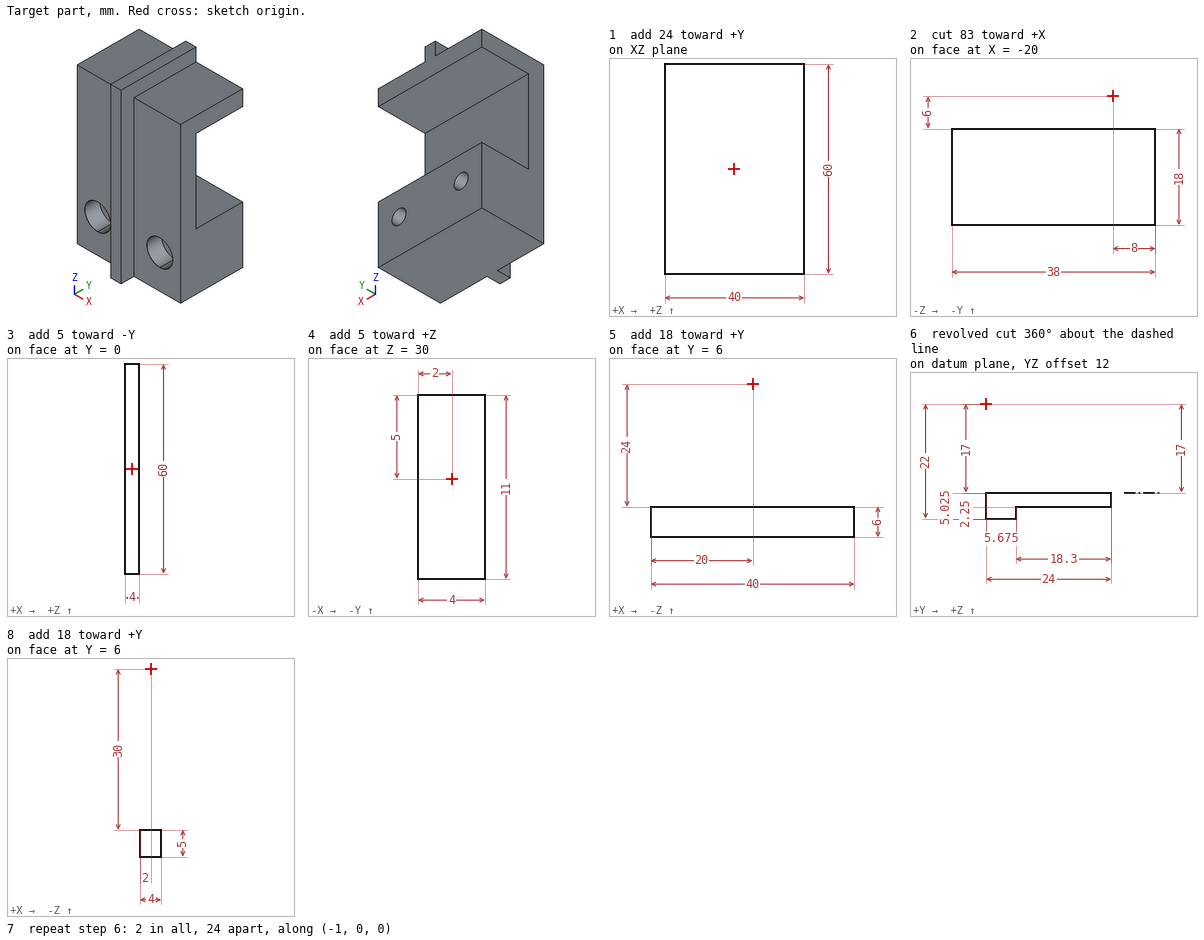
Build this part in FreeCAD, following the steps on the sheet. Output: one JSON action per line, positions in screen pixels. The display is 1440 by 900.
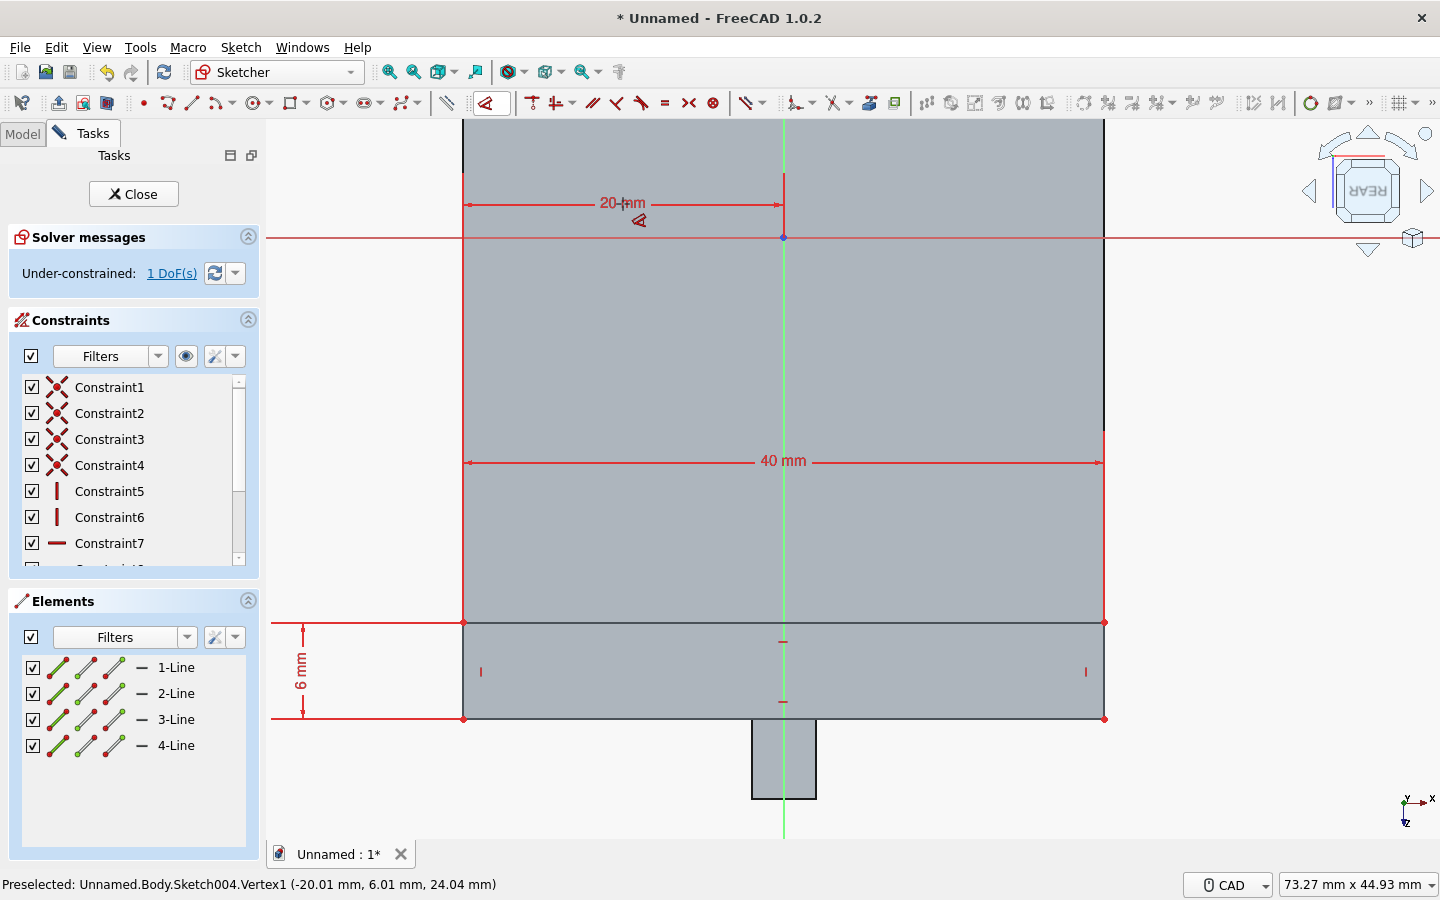
{"action": "left_click", "coordinate": [463, 623]}
{"action": "left_click", "coordinate": [429, 430]}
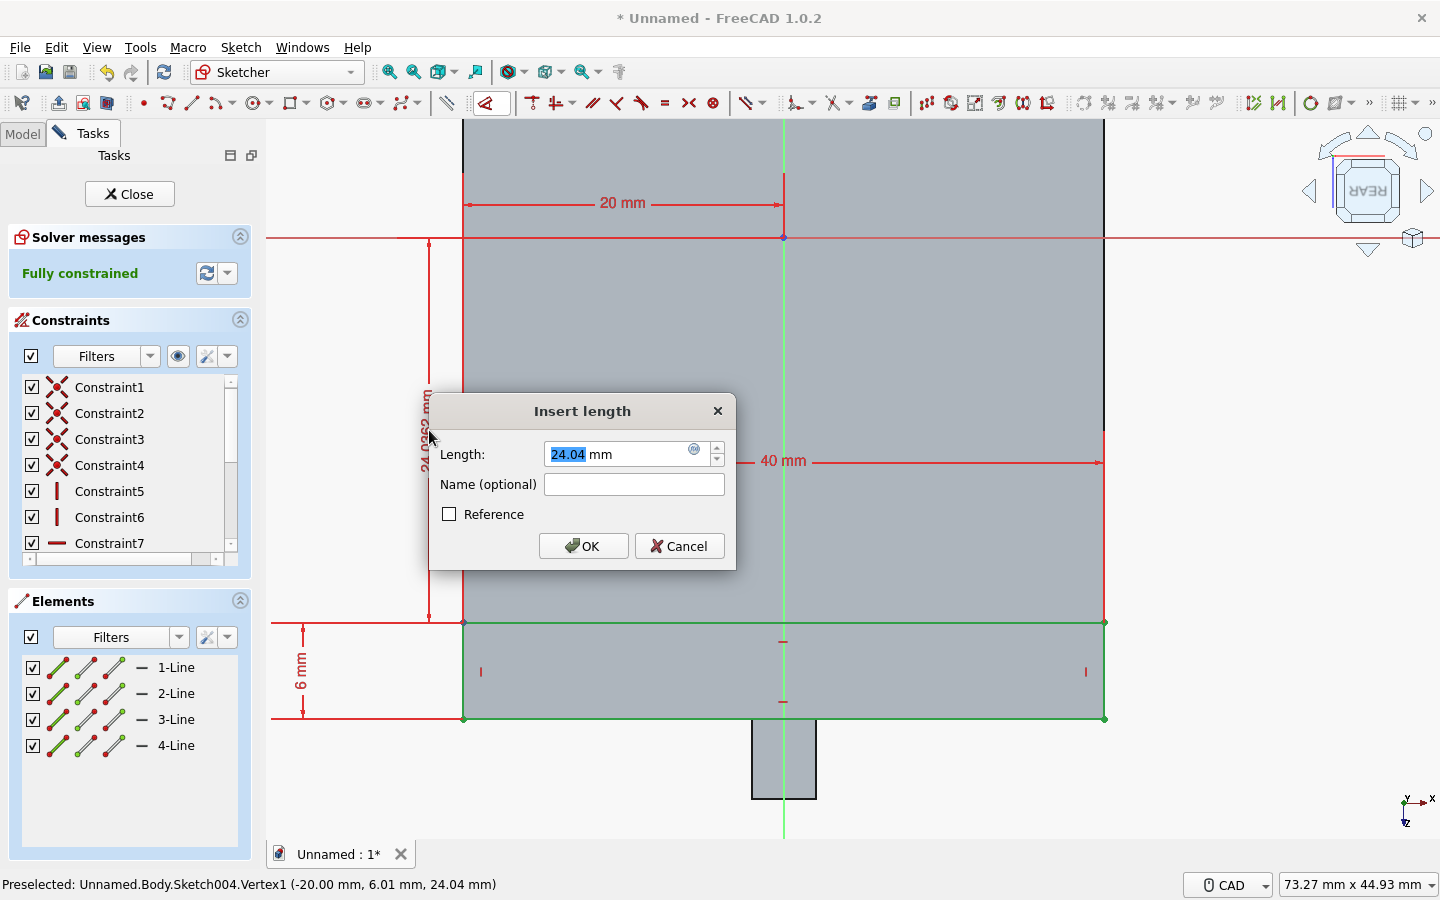
{"action": "type", "text": "24"}
{"action": "key", "text": "Return"}
{"action": "key", "text": "Escape"}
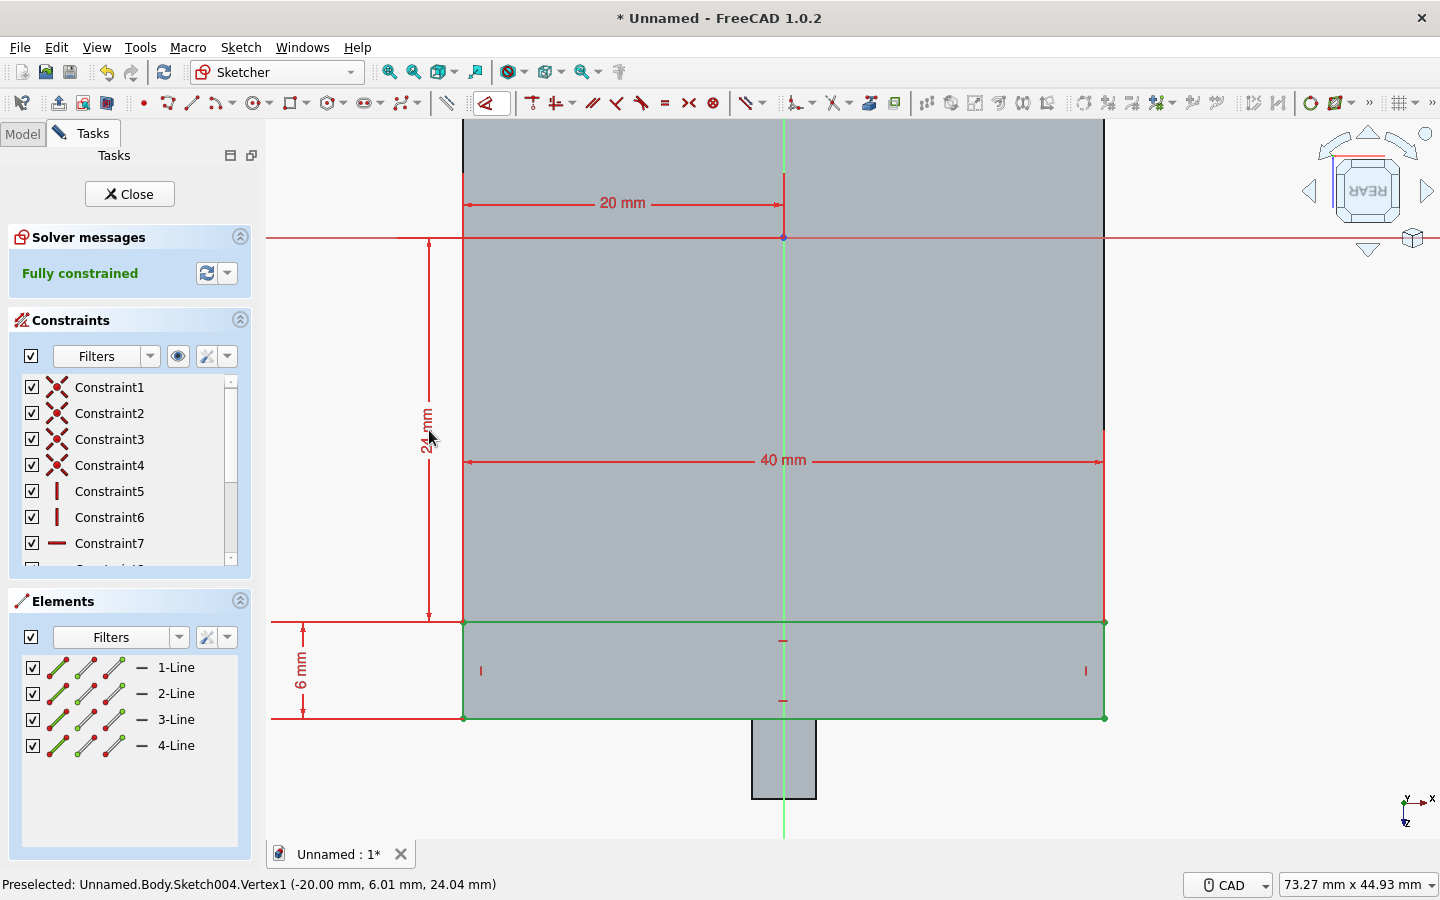
{"action": "left_click", "coordinate": [130, 194]}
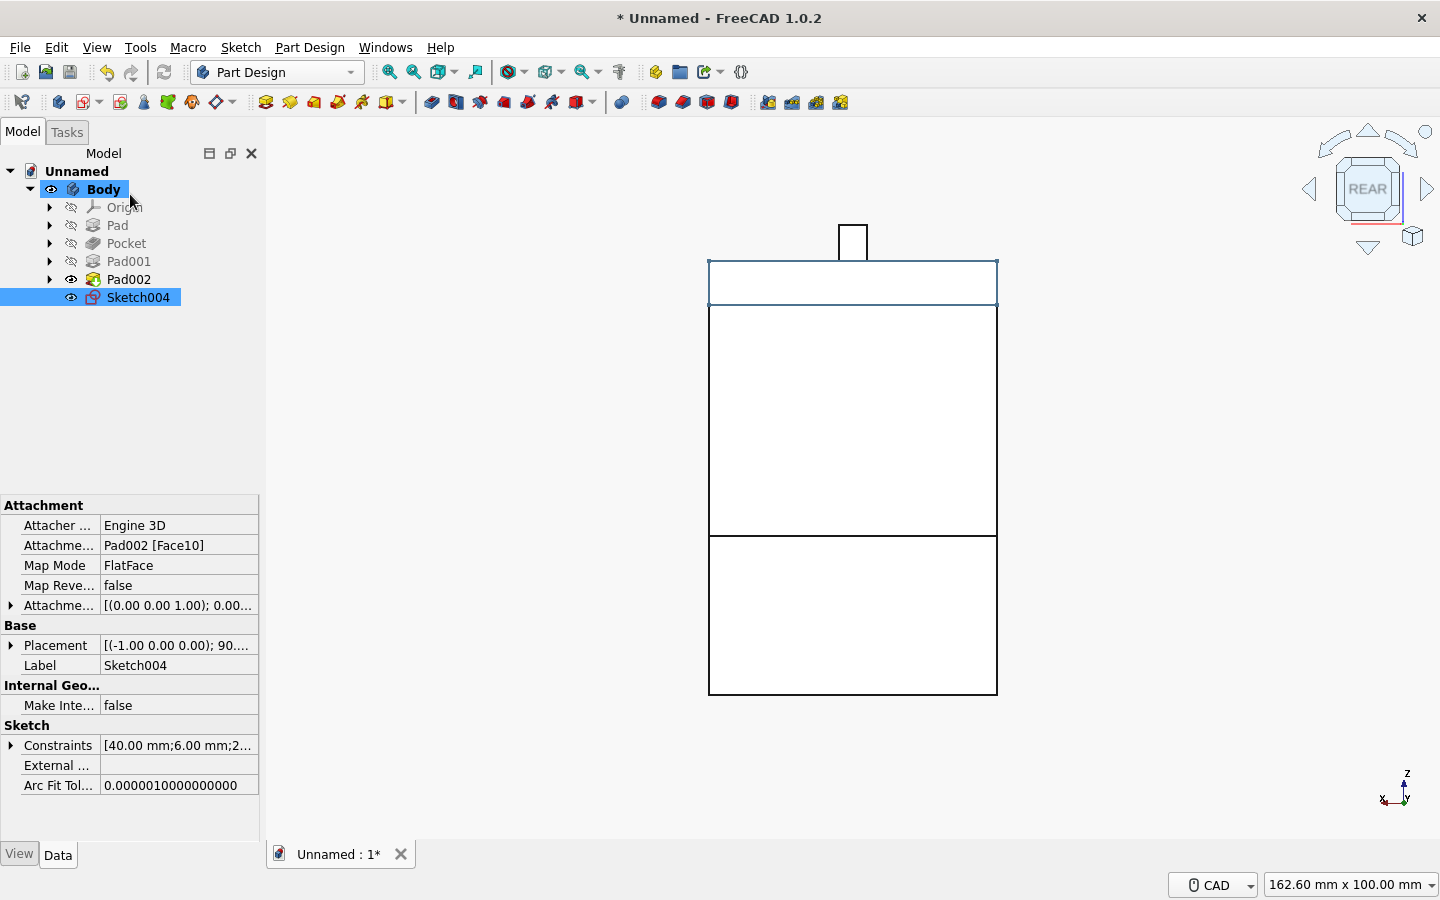
{"action": "left_click", "coordinate": [266, 102]}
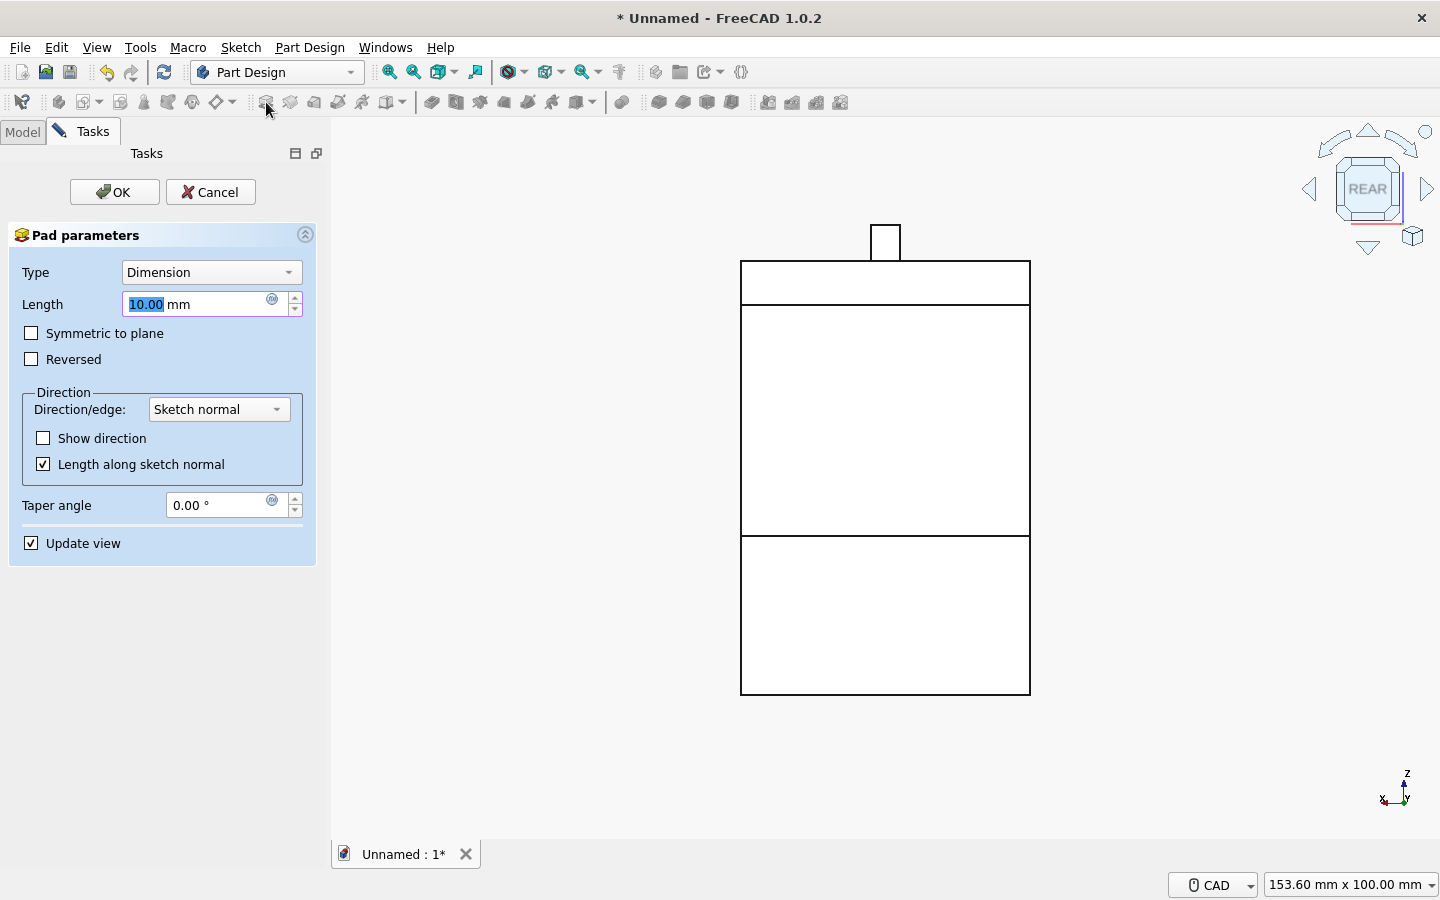
{"action": "type", "text": "18"}
{"action": "key", "text": "Tab"}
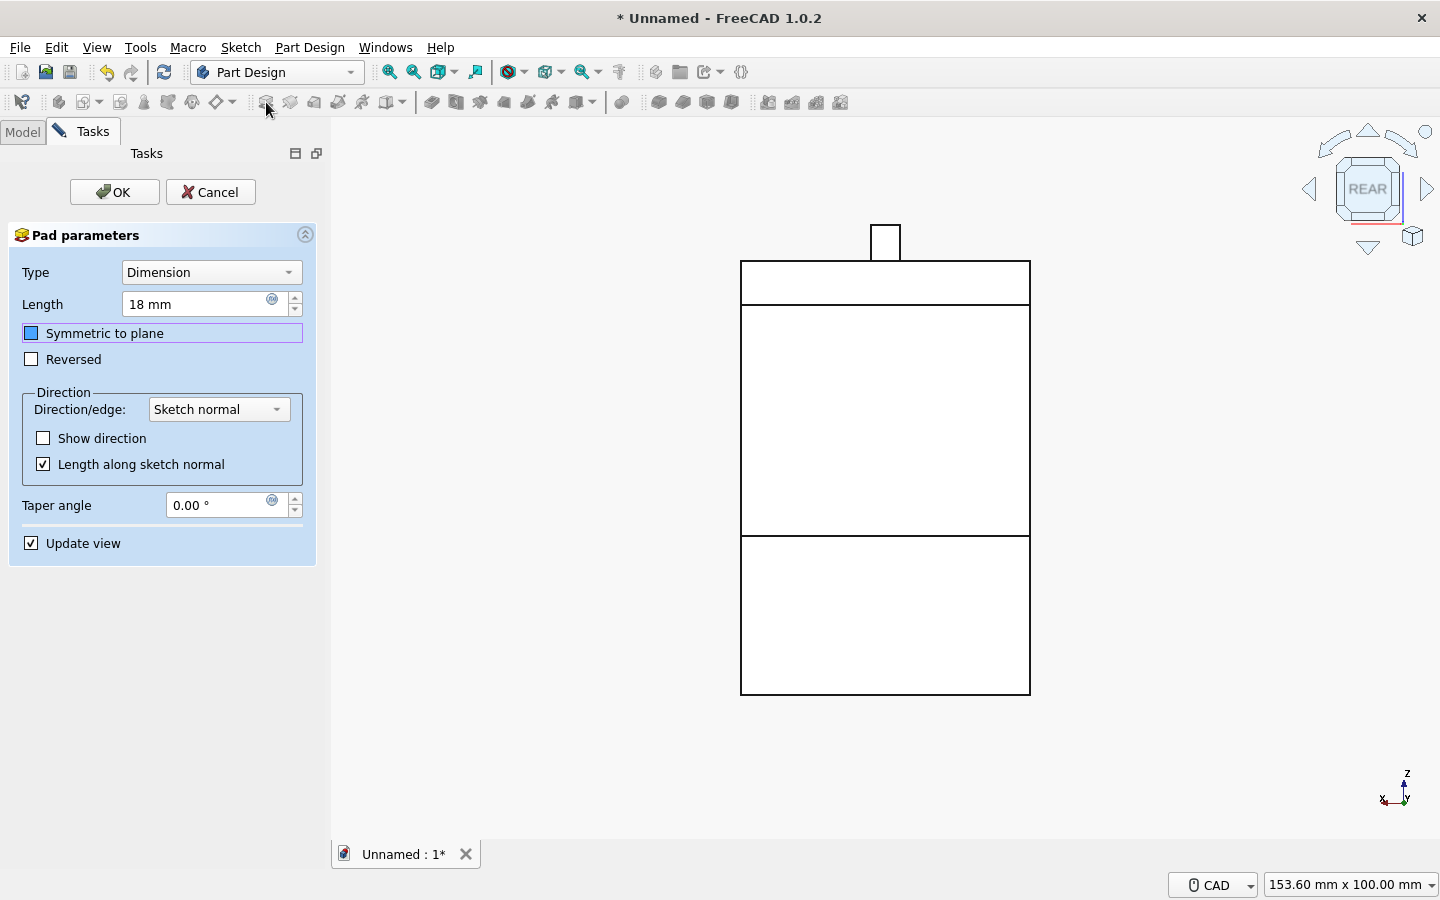
{"action": "left_click", "coordinate": [115, 192]}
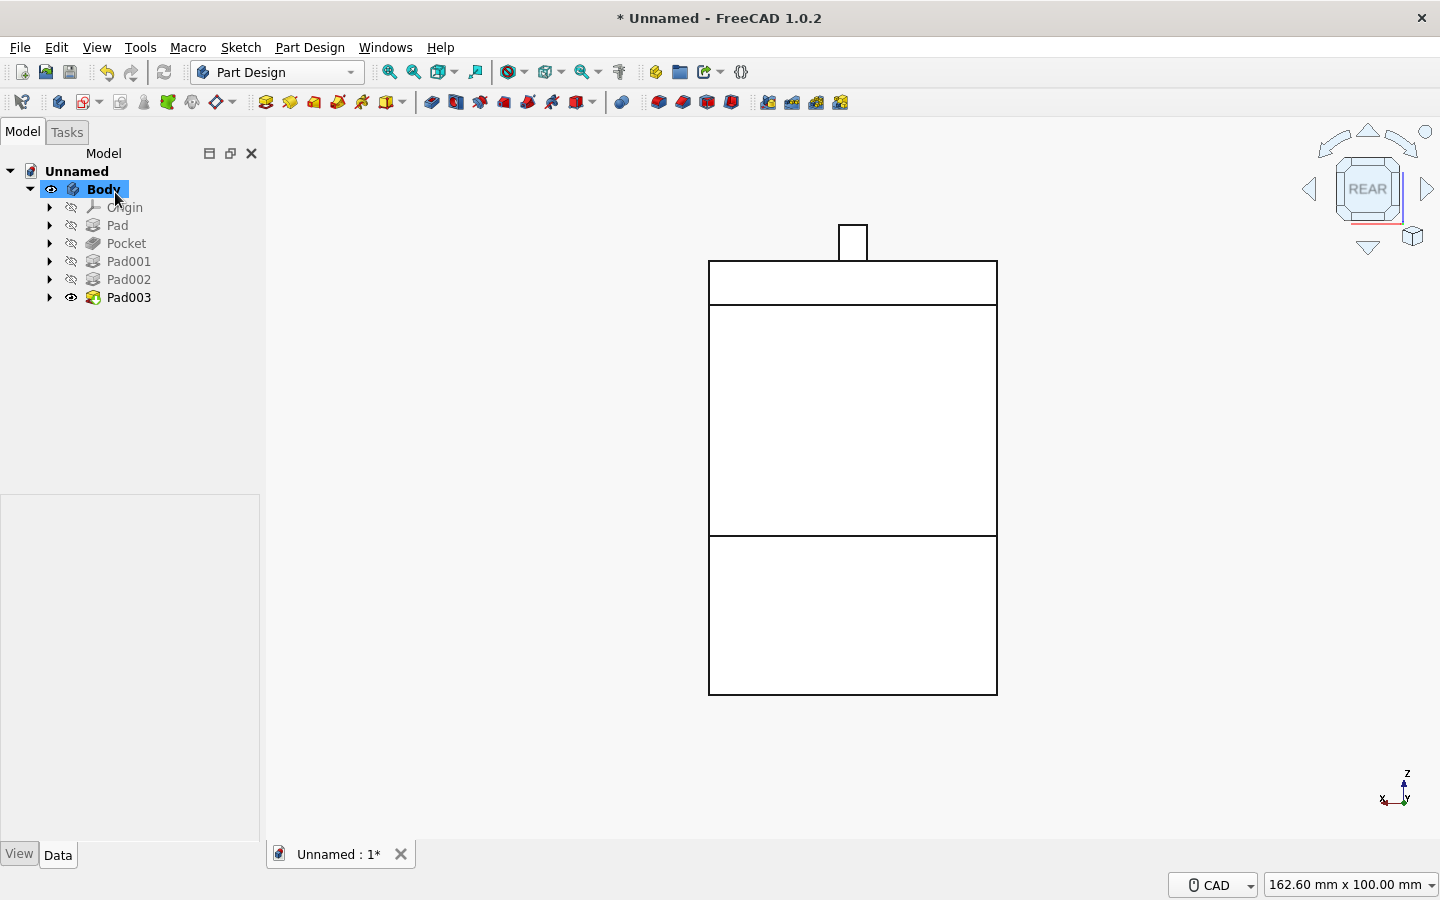
{"action": "left_click", "coordinate": [50, 207]}